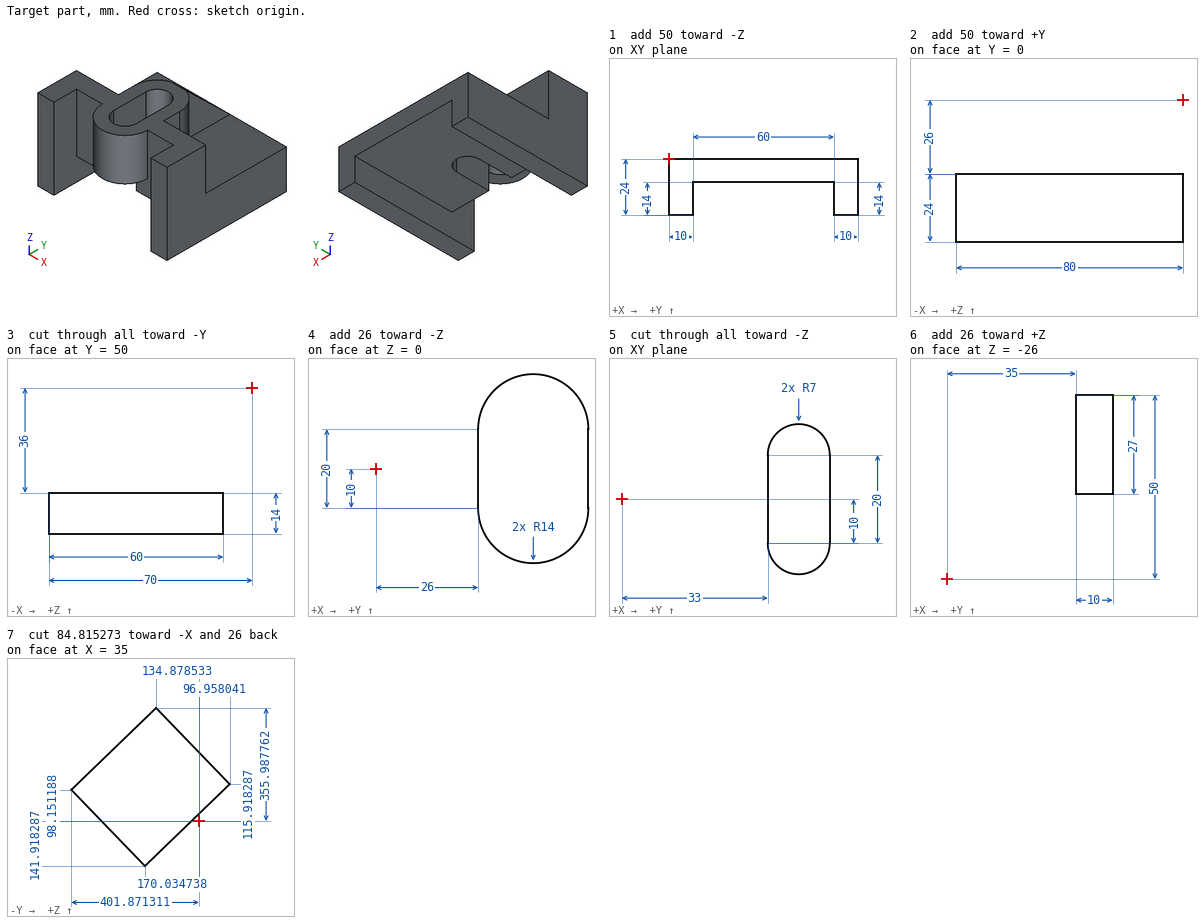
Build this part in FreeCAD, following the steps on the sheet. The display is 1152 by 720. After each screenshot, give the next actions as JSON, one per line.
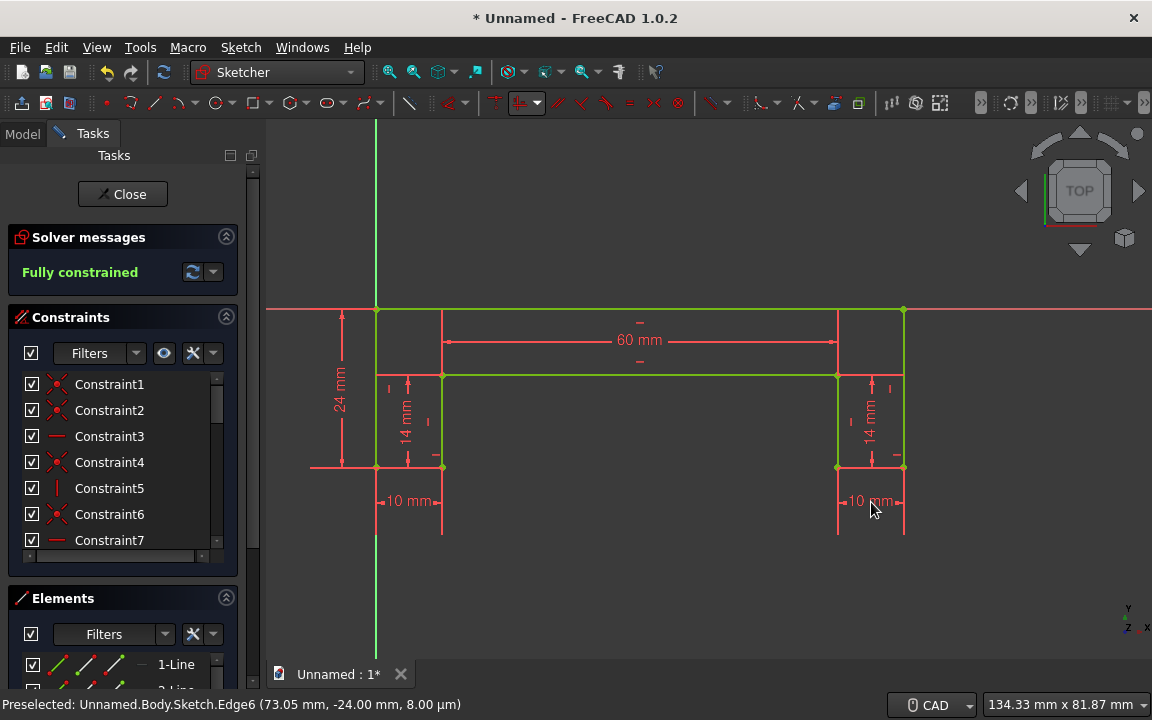
{"action": "left_click", "coordinate": [123, 194]}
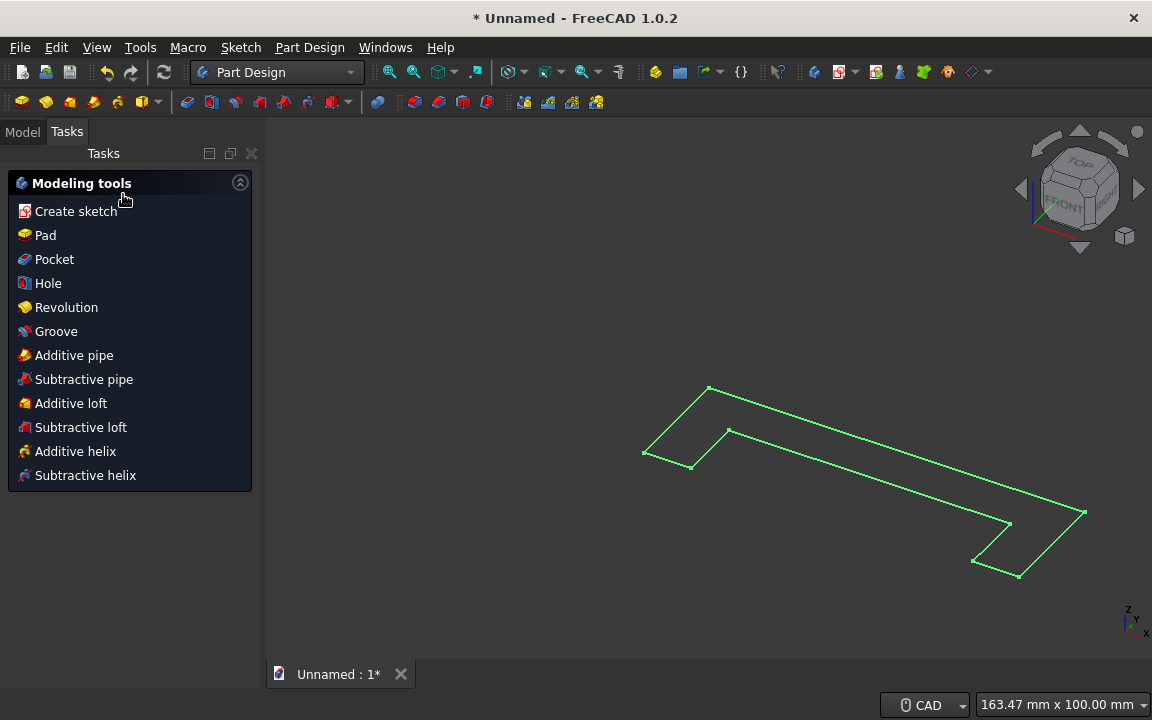
{"action": "left_click", "coordinate": [22, 102]}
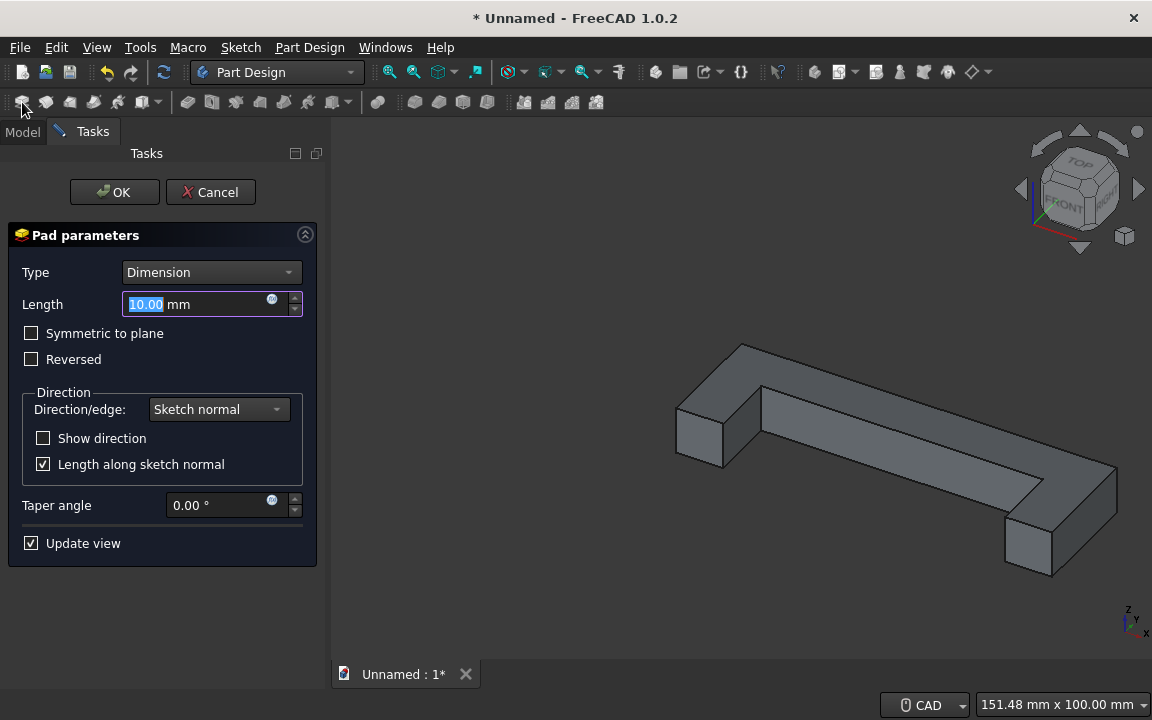
{"action": "type", "text": "50"}
{"action": "key", "text": "Tab"}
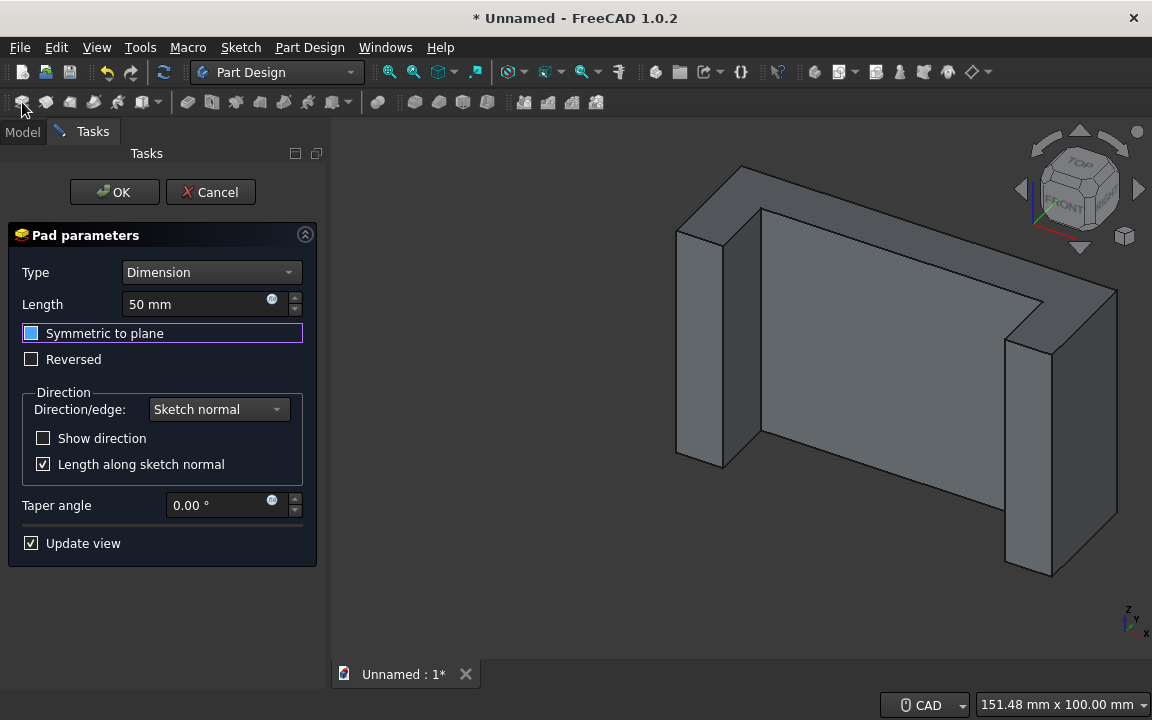
{"action": "left_click", "coordinate": [30, 359]}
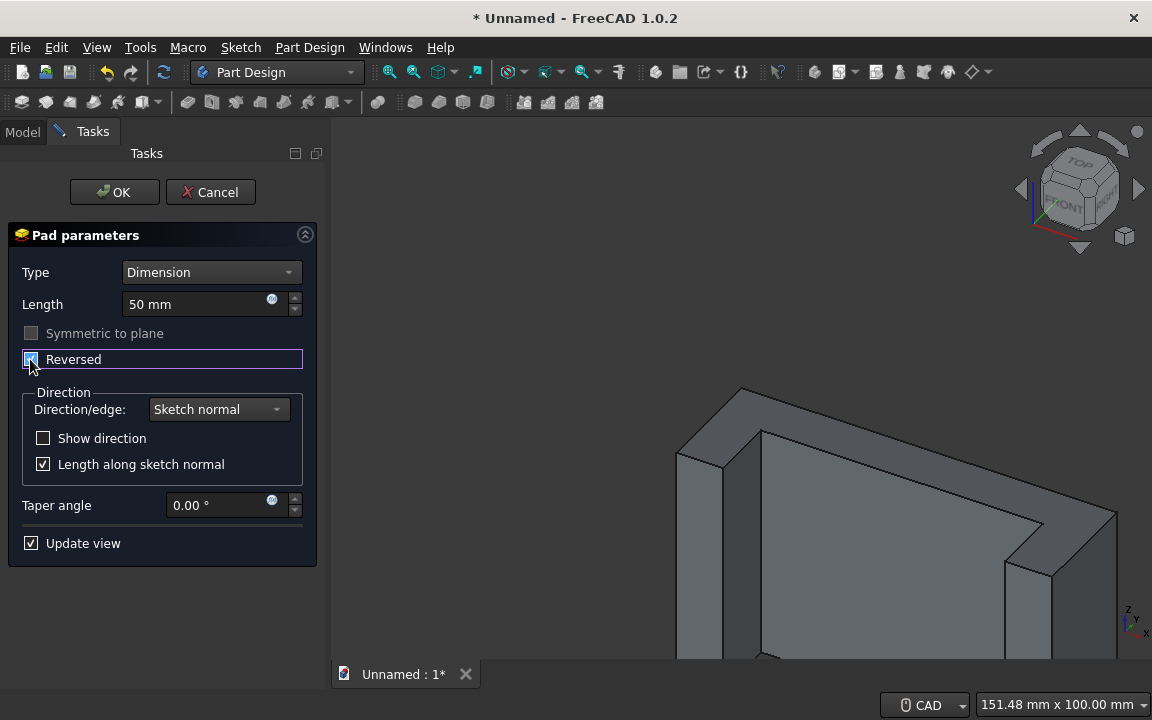
{"action": "left_click", "coordinate": [115, 192]}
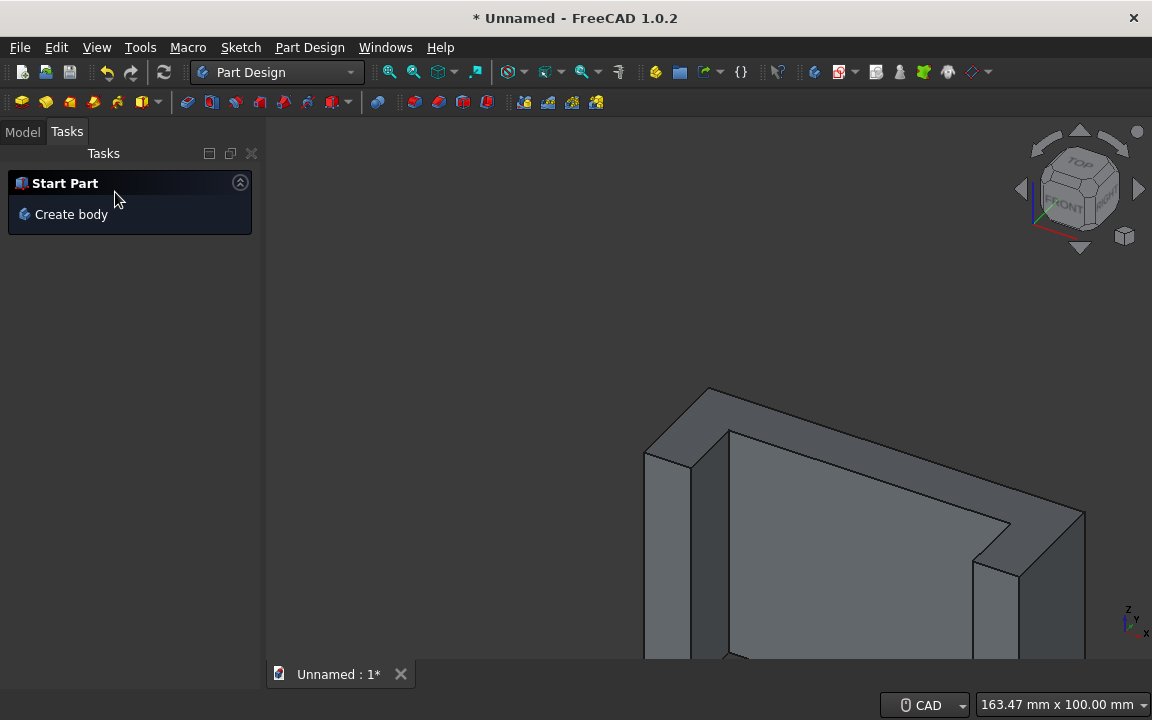
{"action": "left_click", "coordinate": [390, 72]}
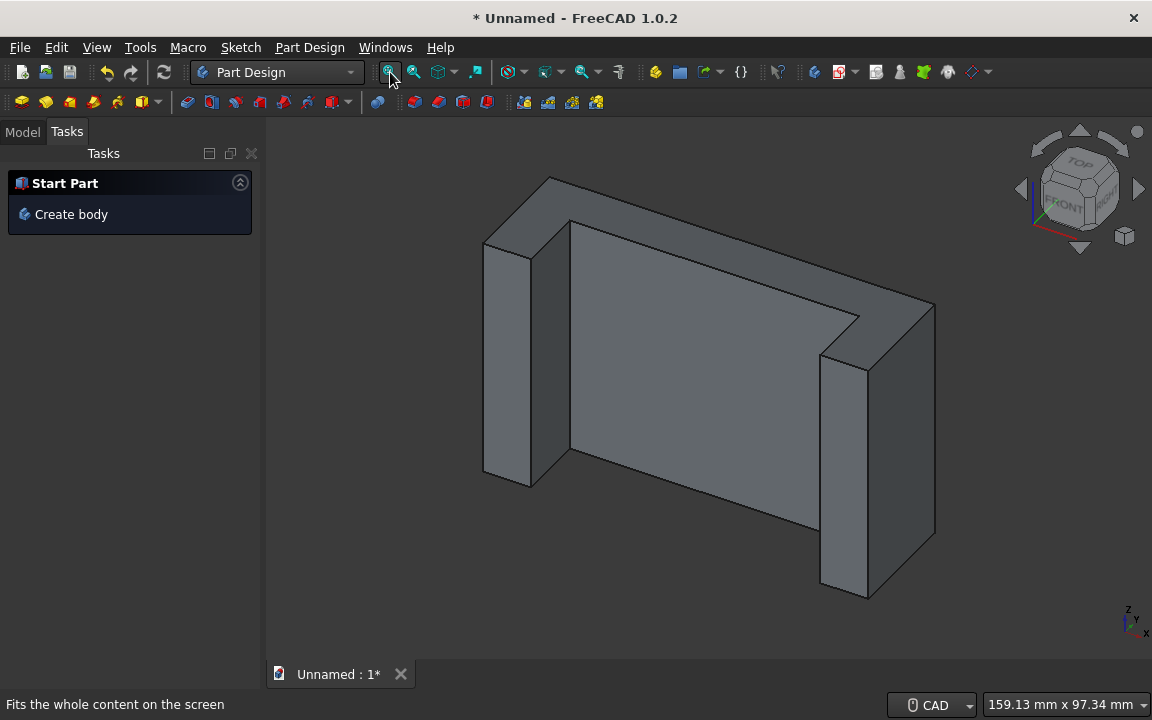
{"action": "key", "text": "4"}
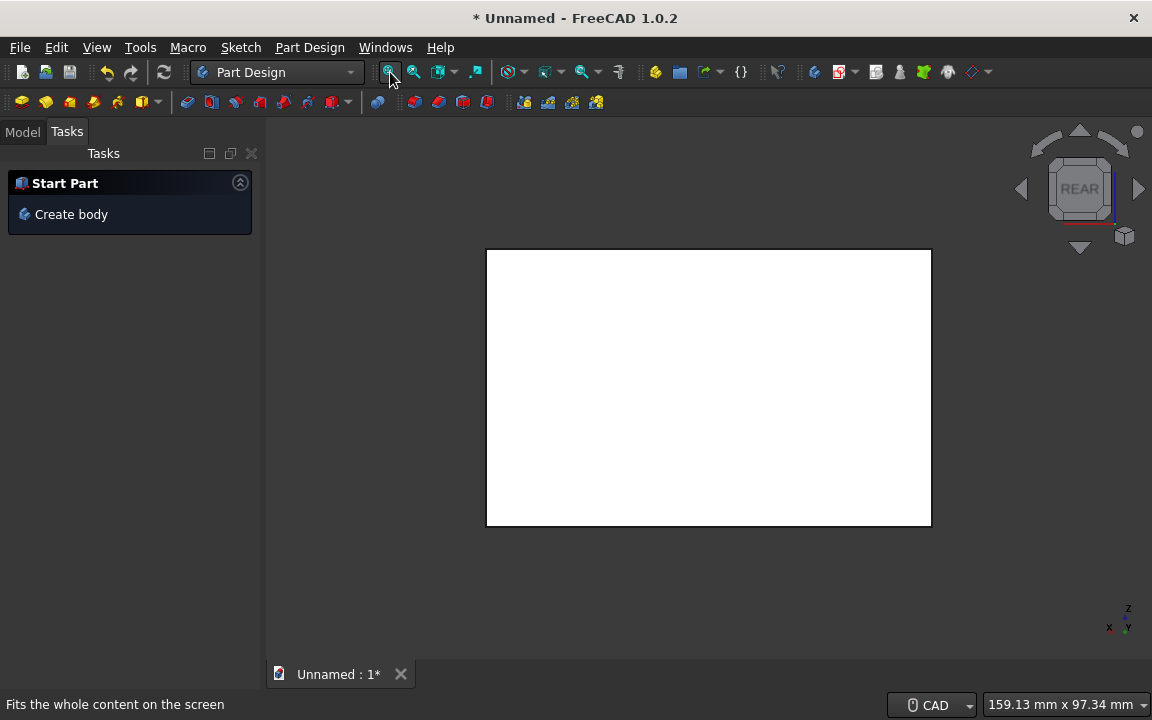
{"action": "left_click", "coordinate": [645, 387]}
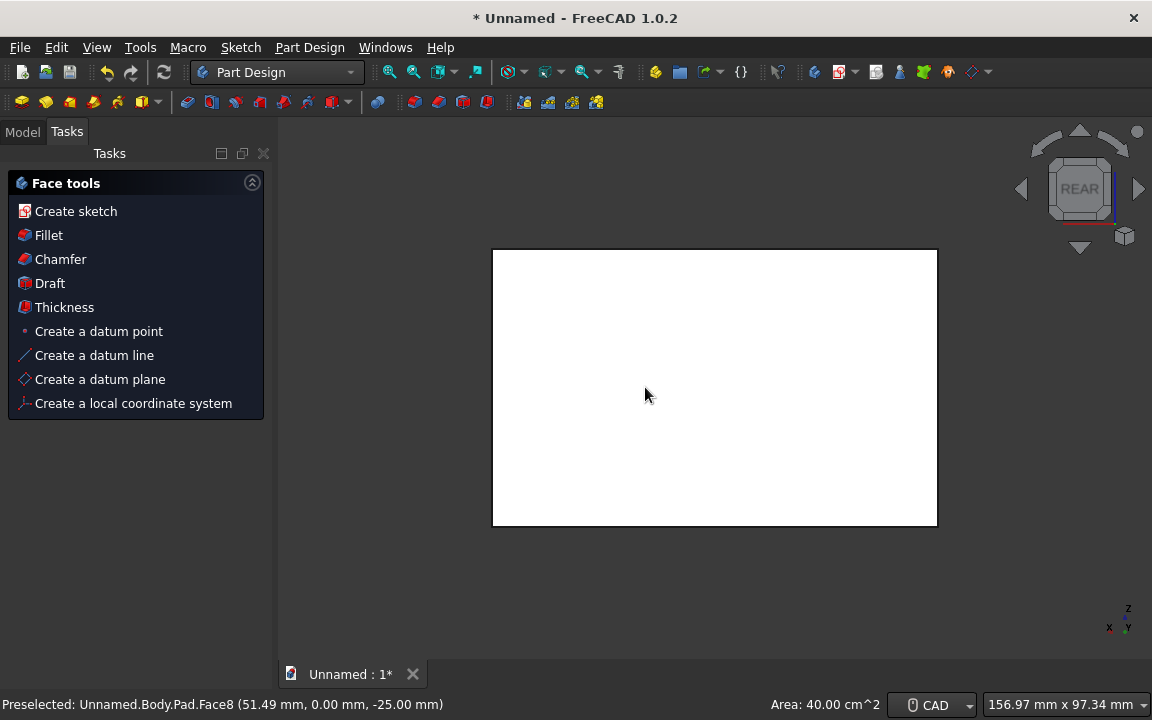
{"action": "left_click", "coordinate": [840, 72]}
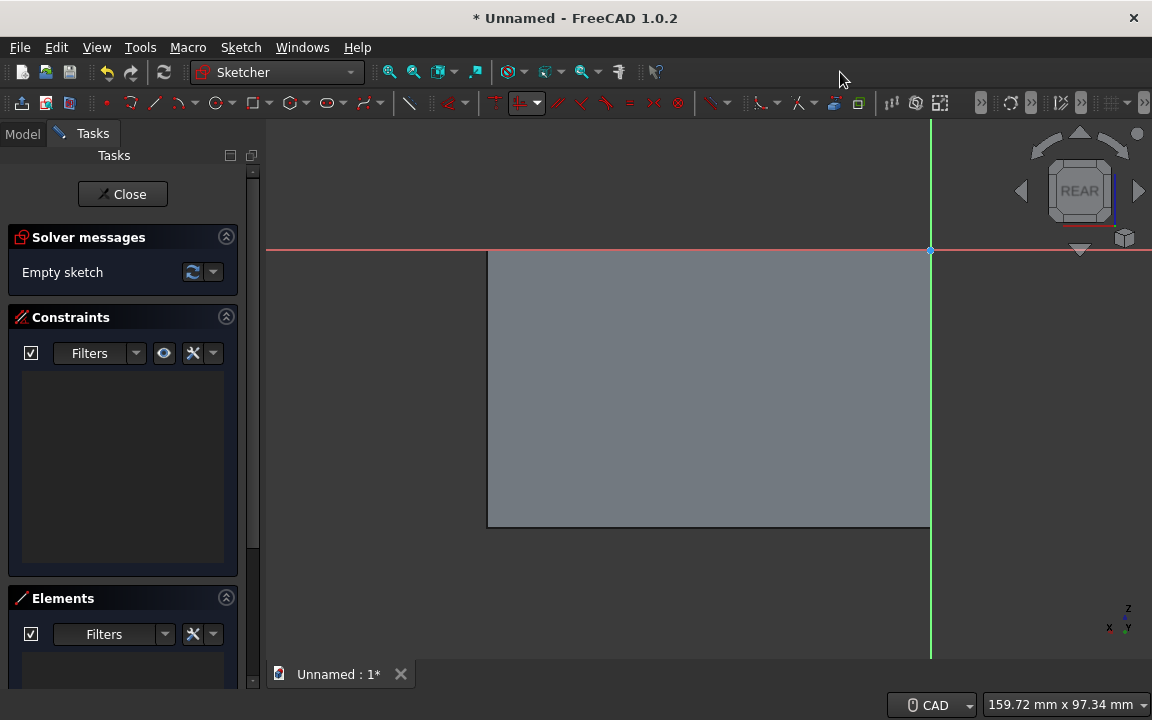
{"action": "left_click", "coordinate": [254, 104]}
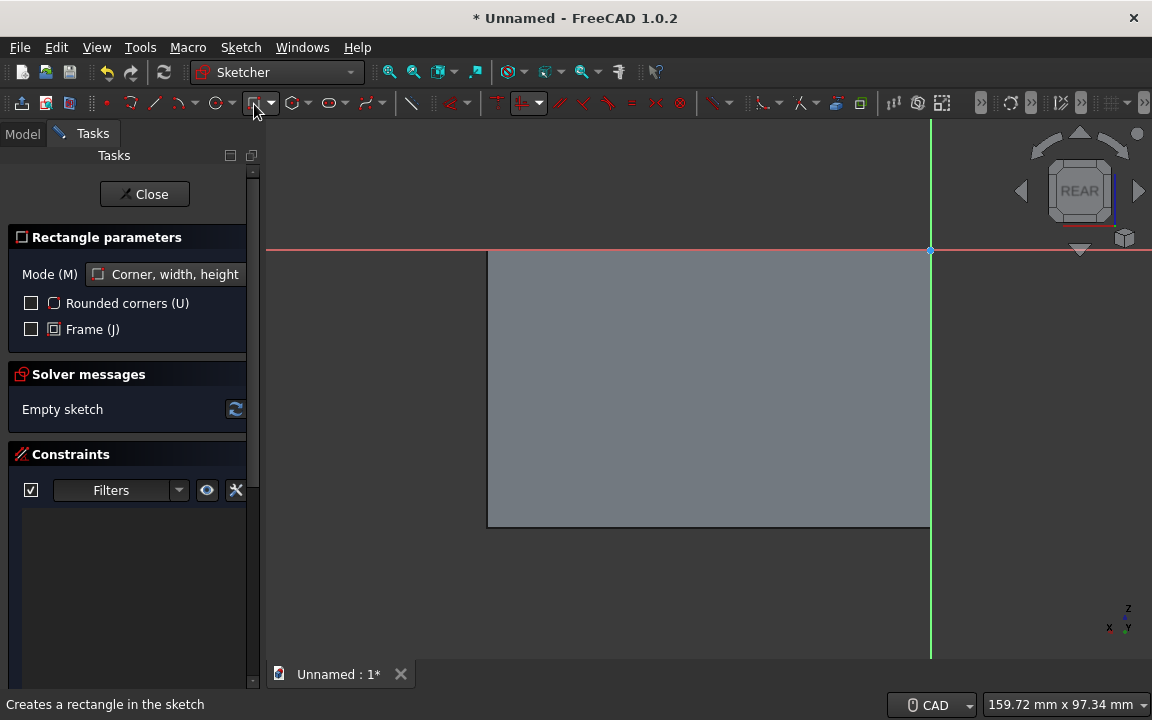
{"action": "left_click", "coordinate": [487, 395]}
{"action": "left_click", "coordinate": [931, 528]}
{"action": "key", "text": "Escape"}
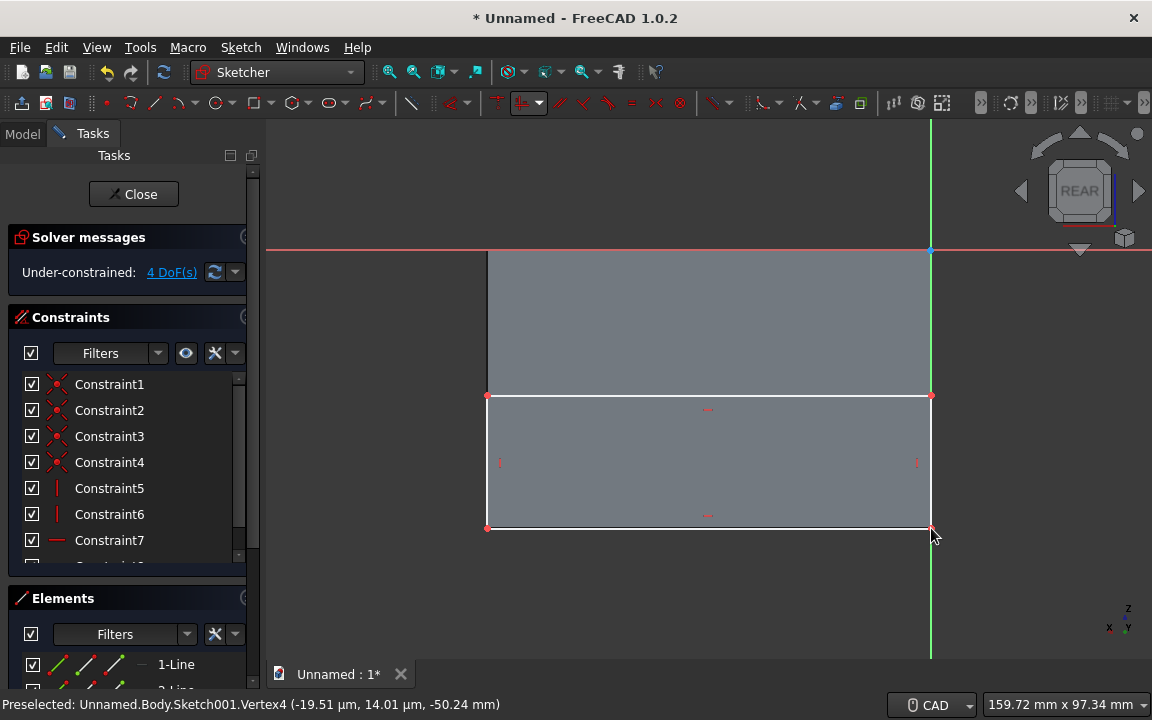
{"action": "left_click", "coordinate": [931, 529]}